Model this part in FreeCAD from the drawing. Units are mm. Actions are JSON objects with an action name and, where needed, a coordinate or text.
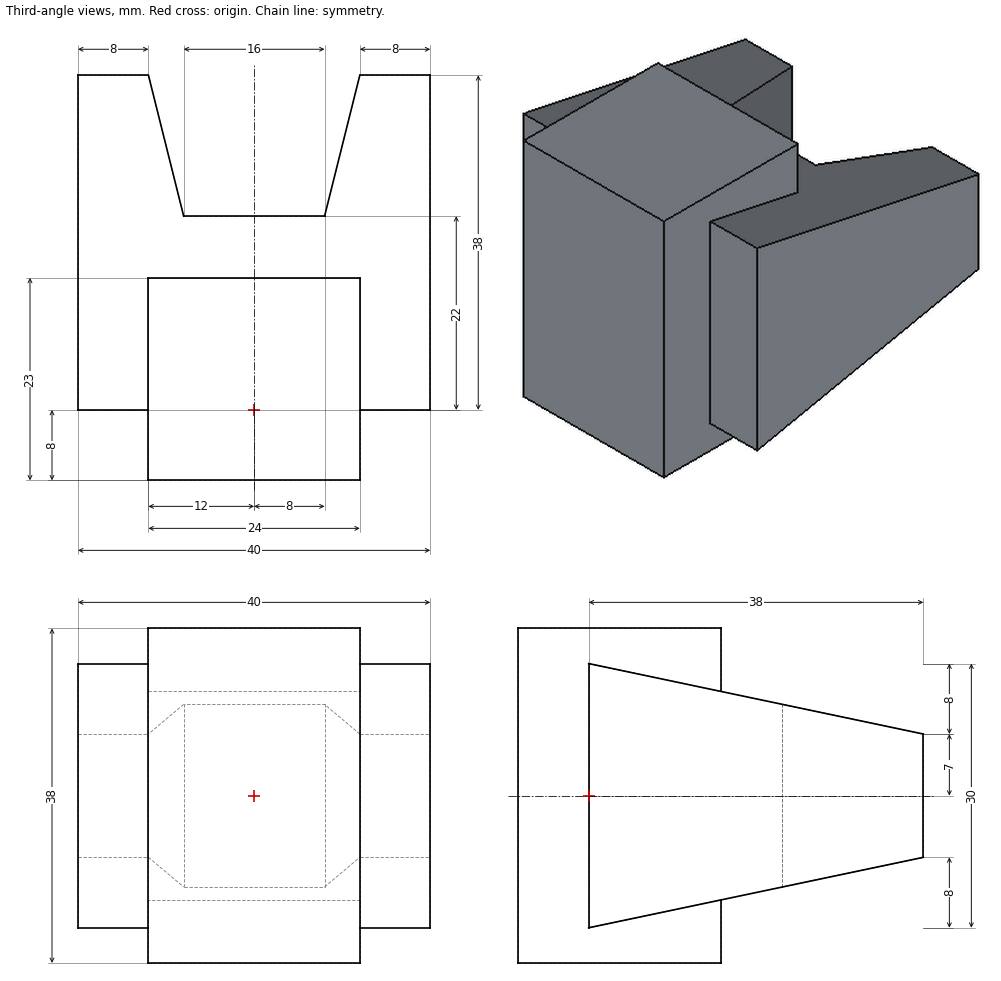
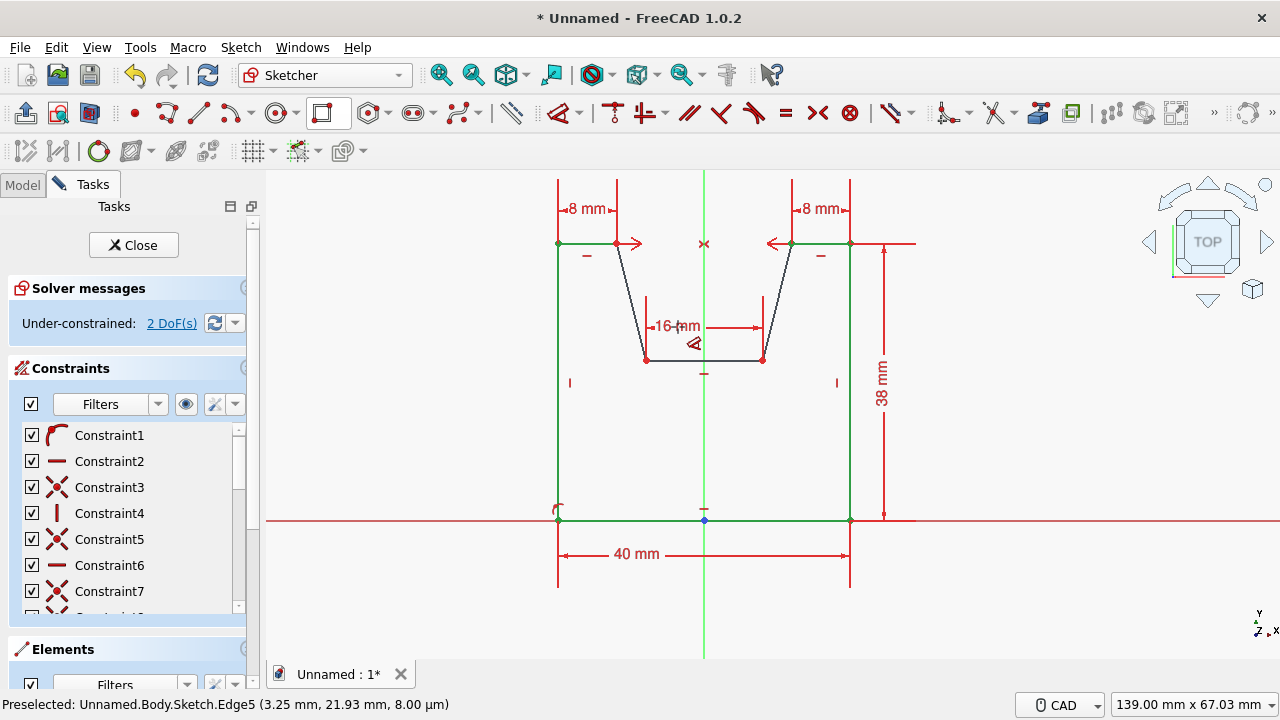
{"action": "left_click", "coordinate": [763, 361]}
{"action": "left_click", "coordinate": [734, 555]}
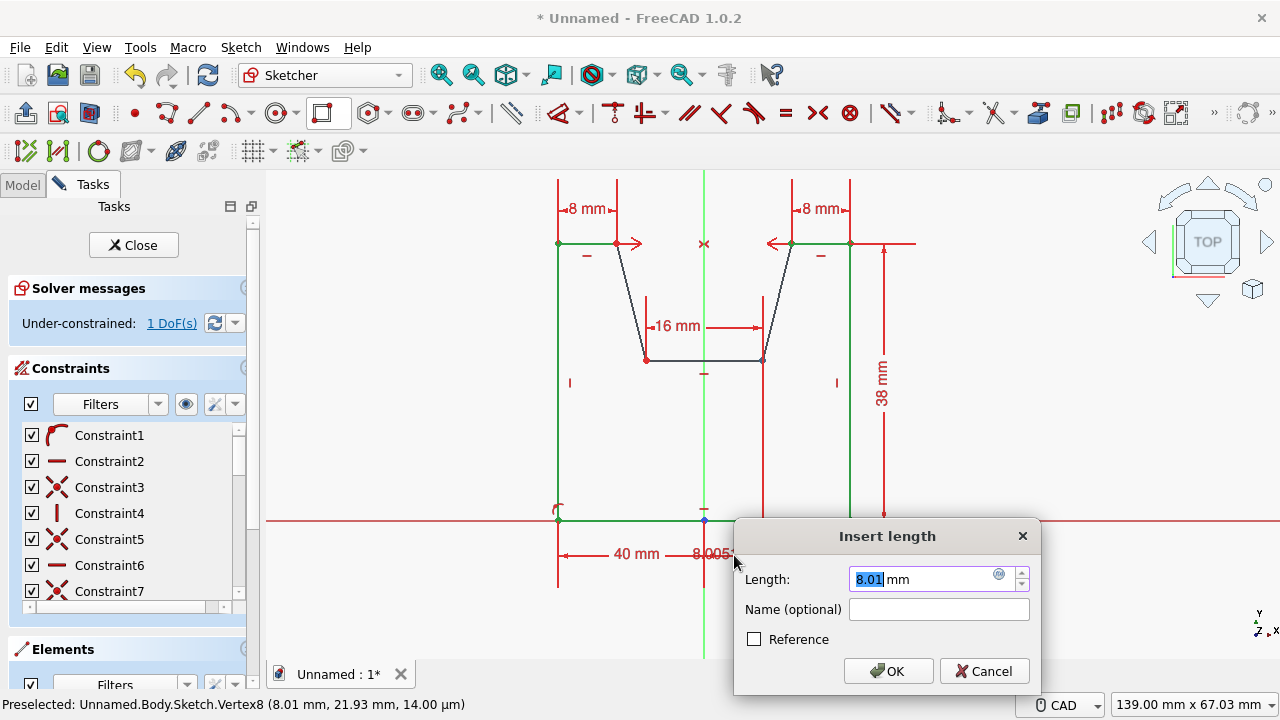
{"action": "type", "text": "8"}
{"action": "key", "text": "Return"}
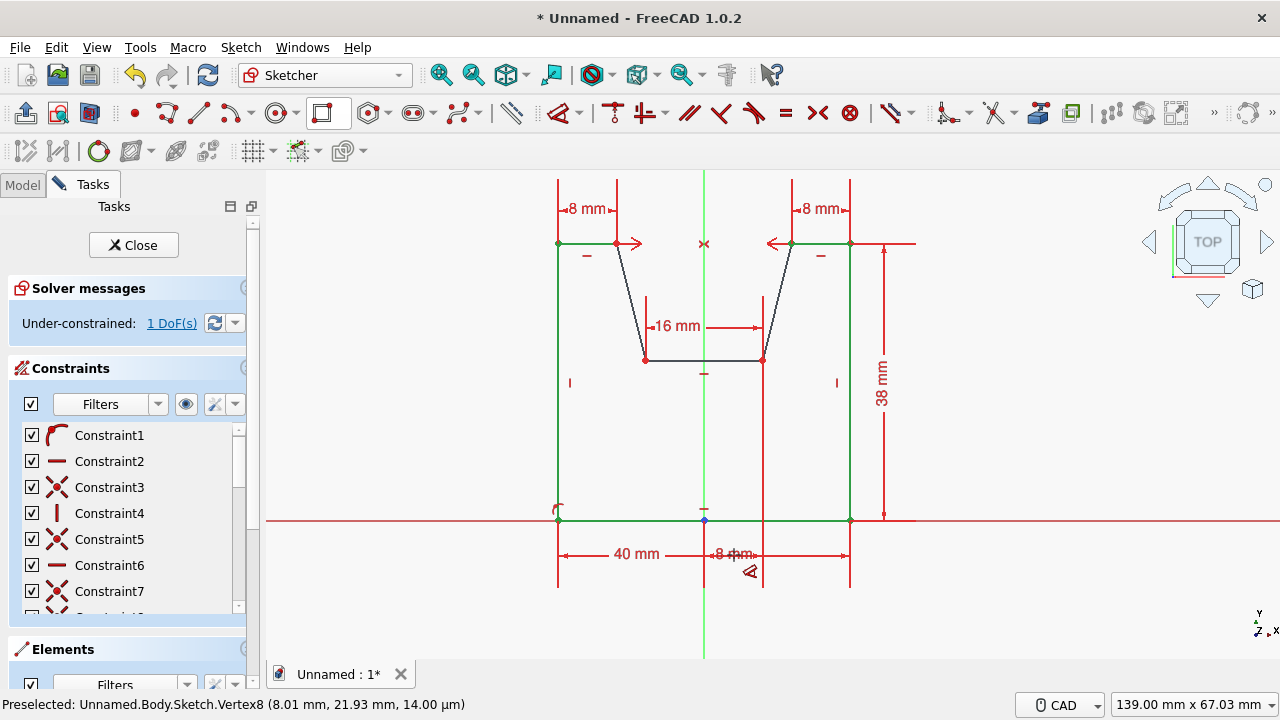
{"action": "left_click", "coordinate": [763, 361]}
{"action": "left_click", "coordinate": [797, 441]}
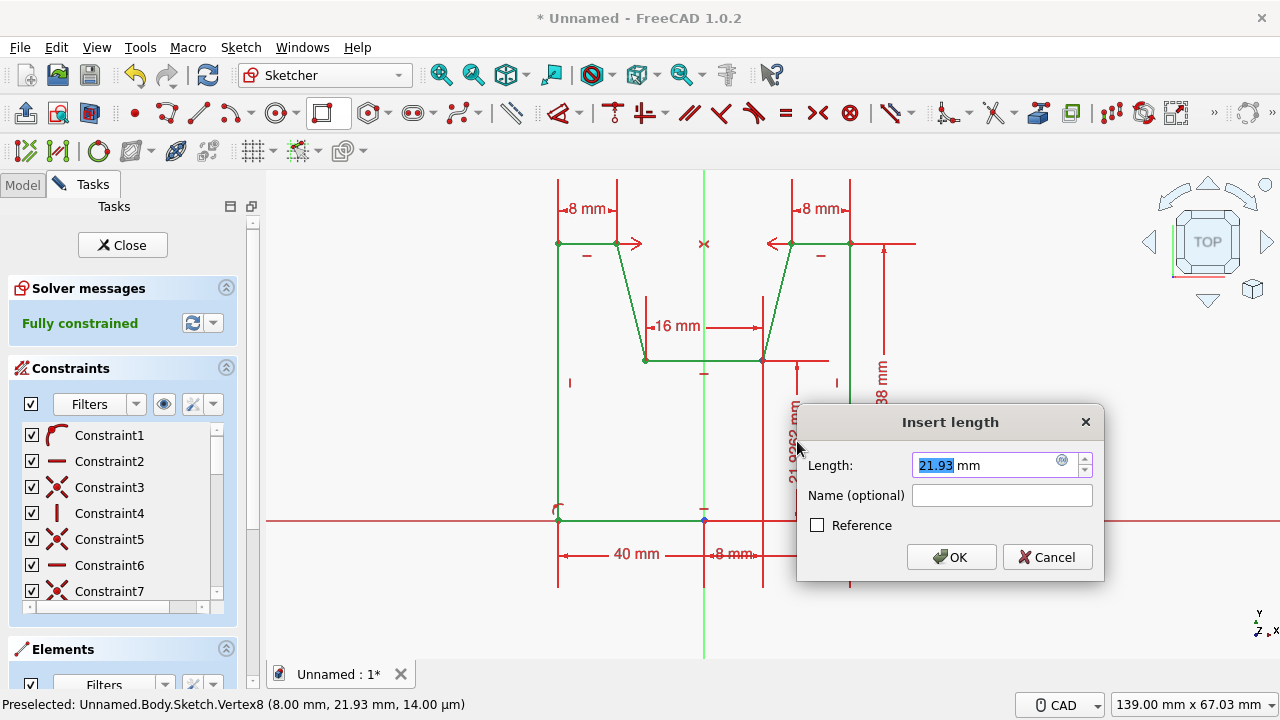
{"action": "type", "text": "22"}
{"action": "key", "text": "Return"}
{"action": "key", "text": "Escape"}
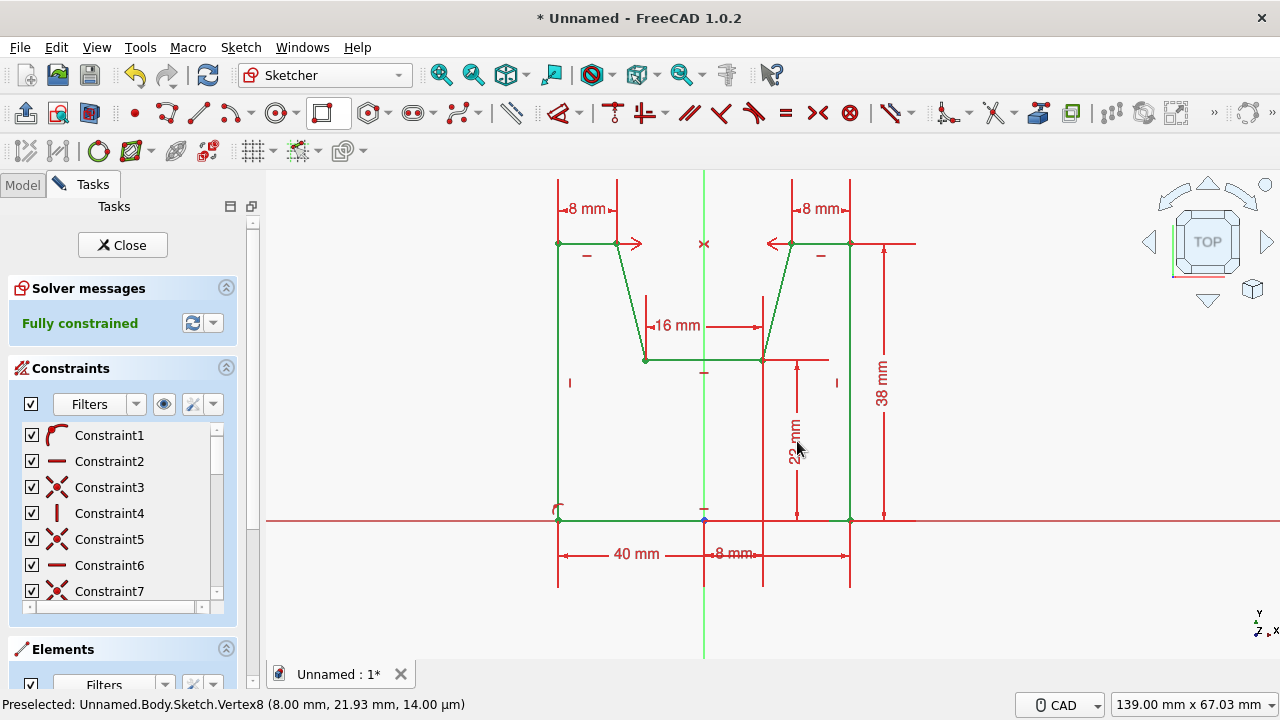
{"action": "left_click", "coordinate": [123, 245]}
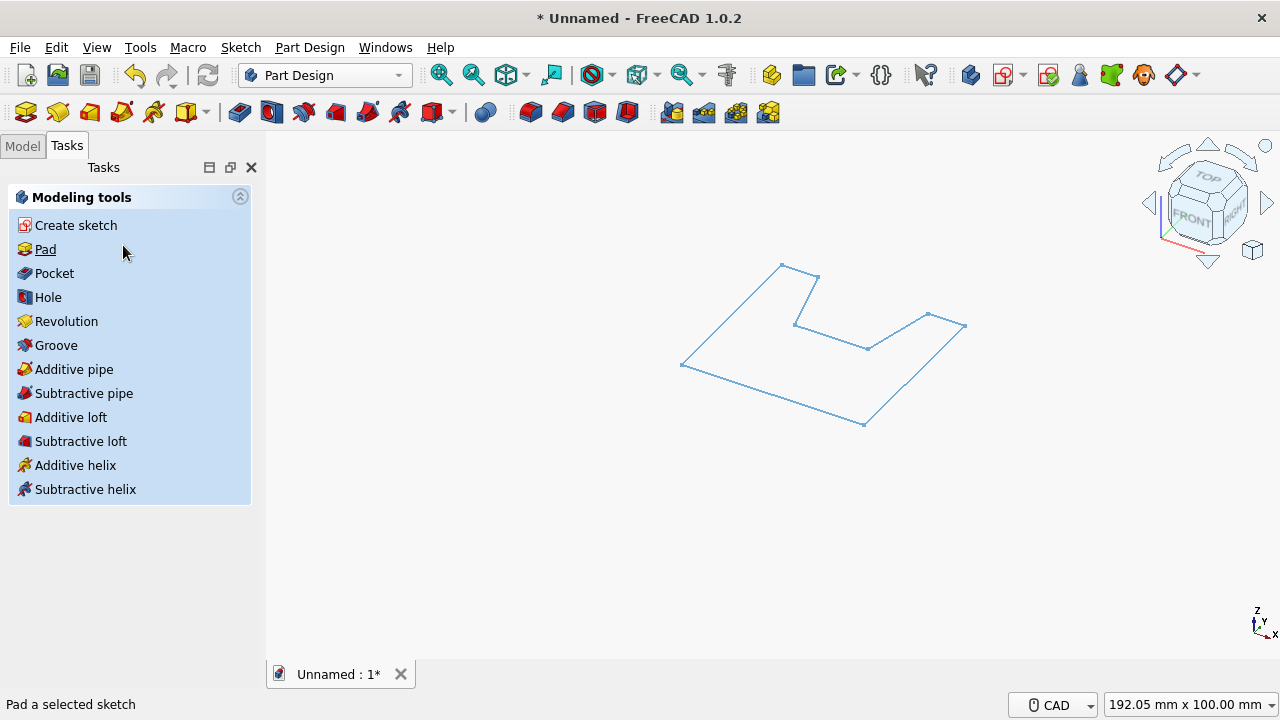
{"action": "left_click", "coordinate": [26, 112]}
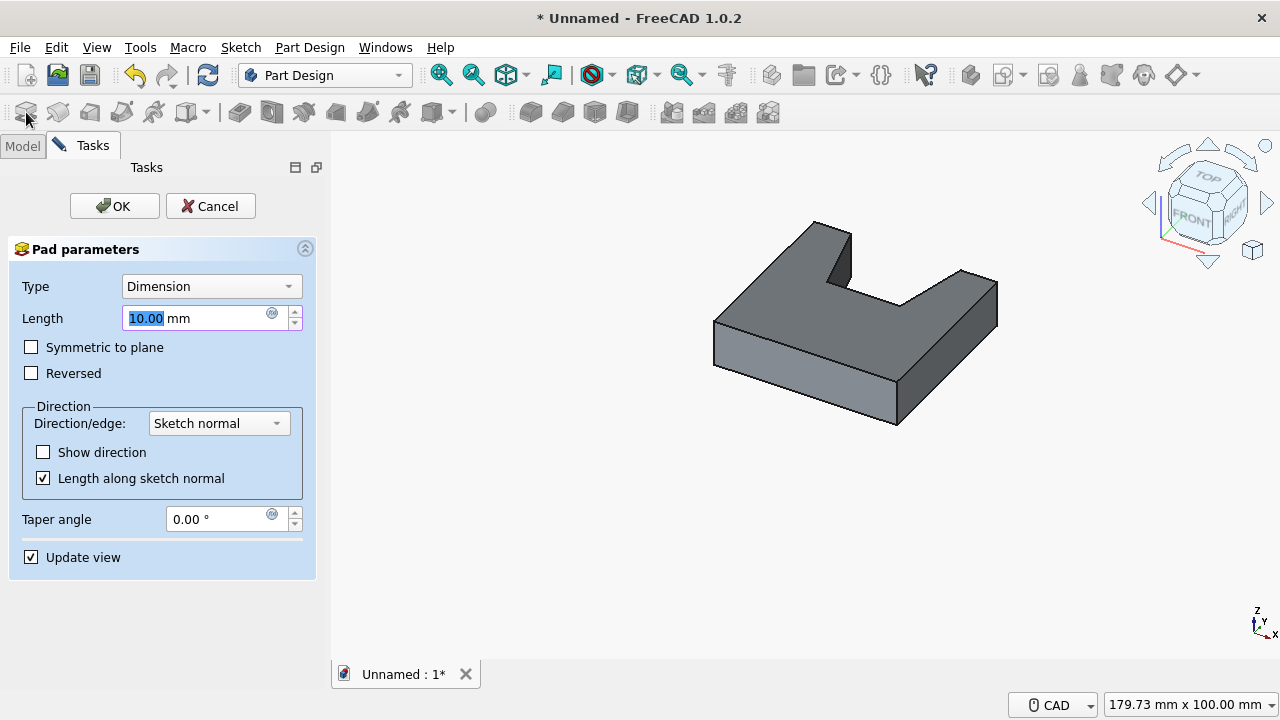
{"action": "type", "text": "30"}
{"action": "key", "text": "Tab"}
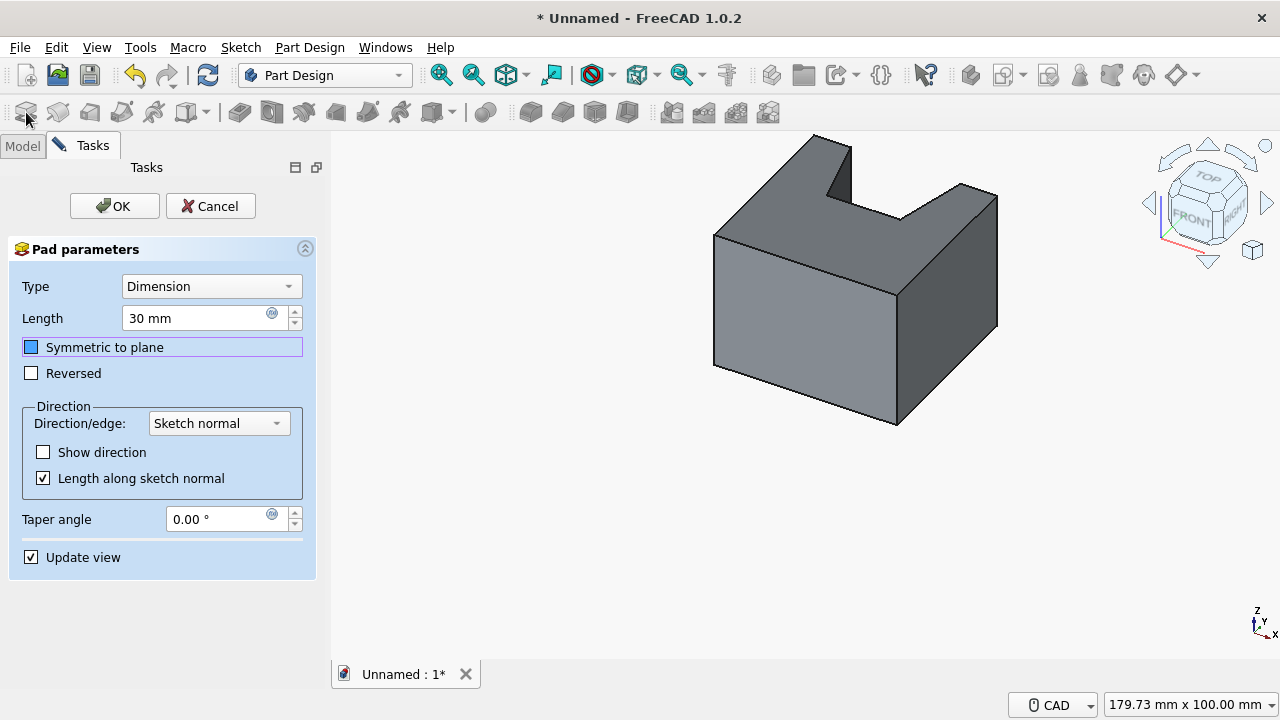
{"action": "left_click", "coordinate": [30, 347]}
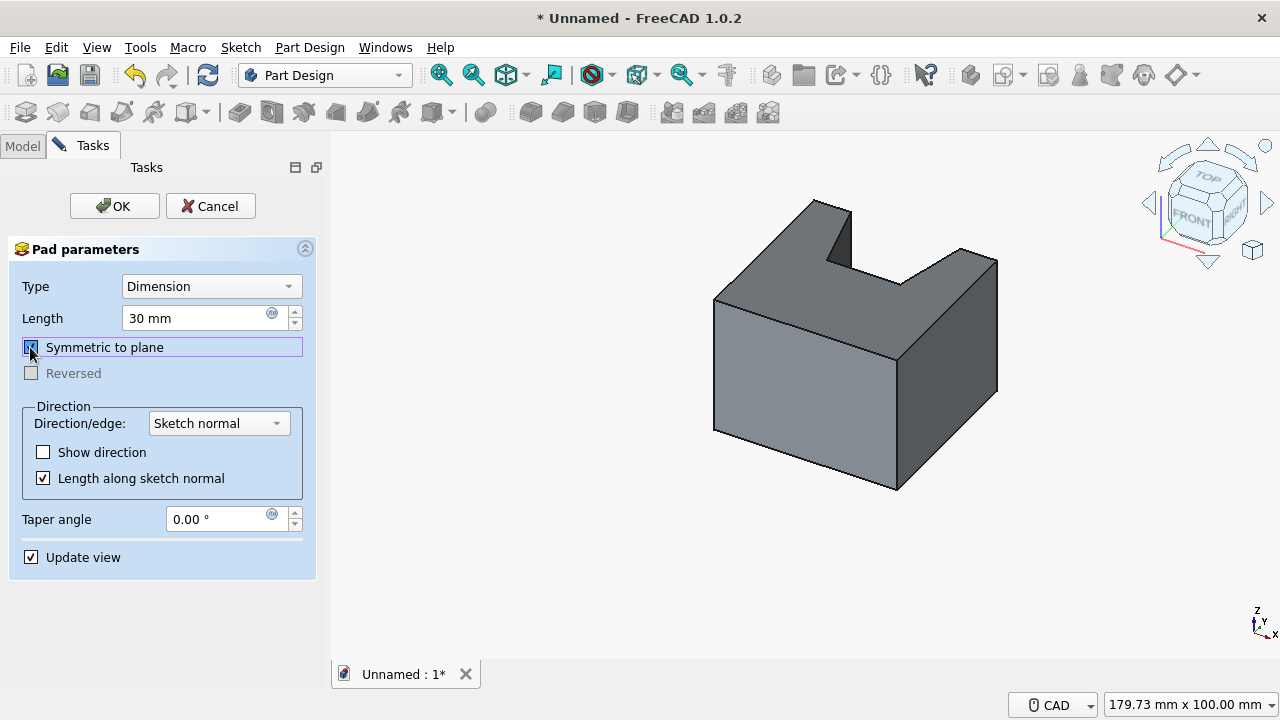
{"action": "left_click", "coordinate": [115, 206]}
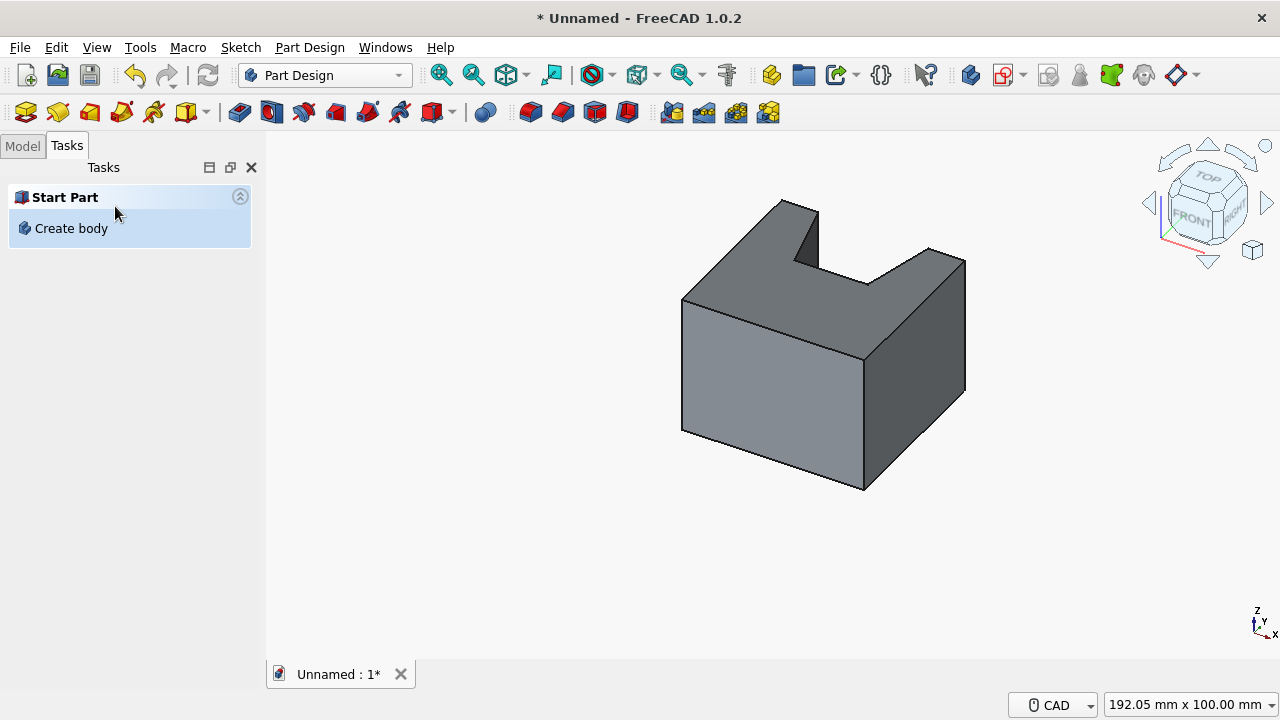
{"action": "left_click", "coordinate": [1004, 76]}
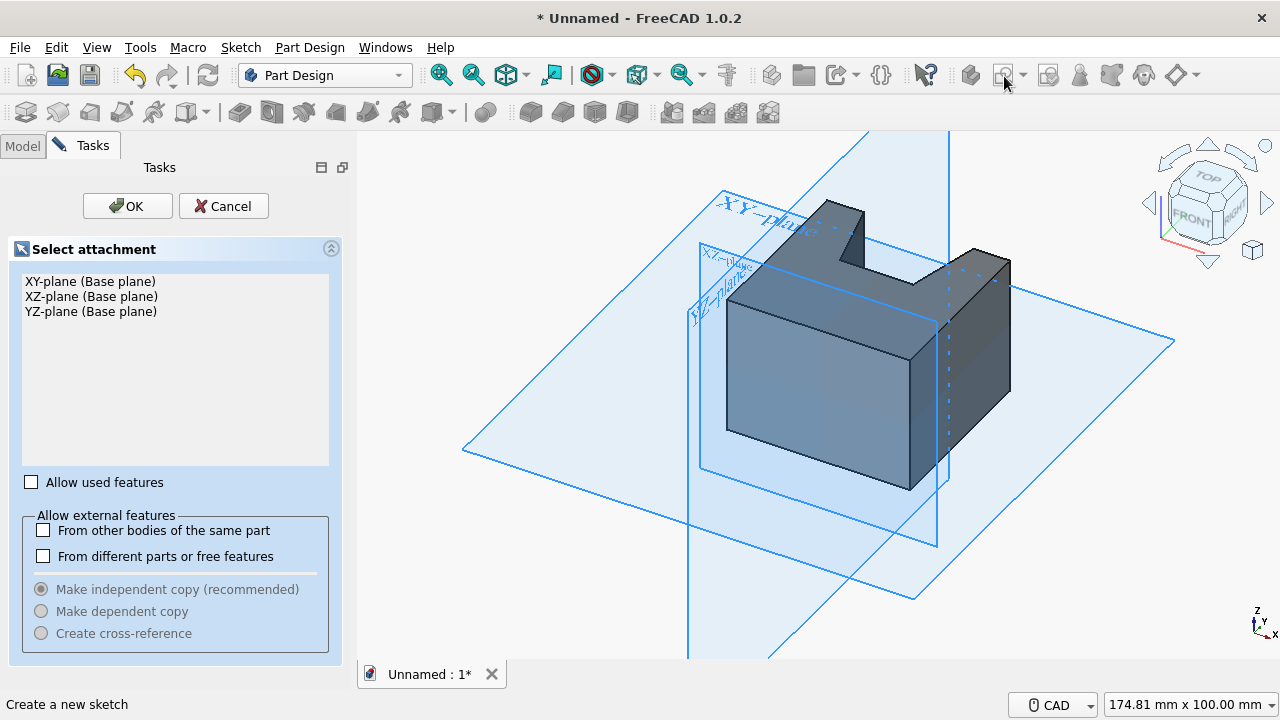
{"action": "left_click", "coordinate": [82, 312]}